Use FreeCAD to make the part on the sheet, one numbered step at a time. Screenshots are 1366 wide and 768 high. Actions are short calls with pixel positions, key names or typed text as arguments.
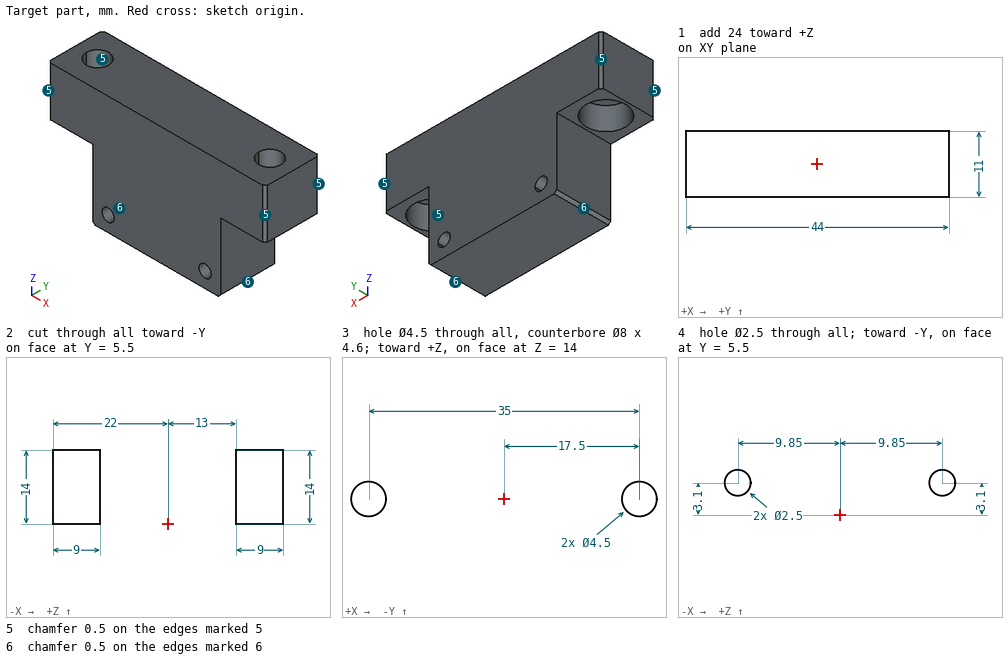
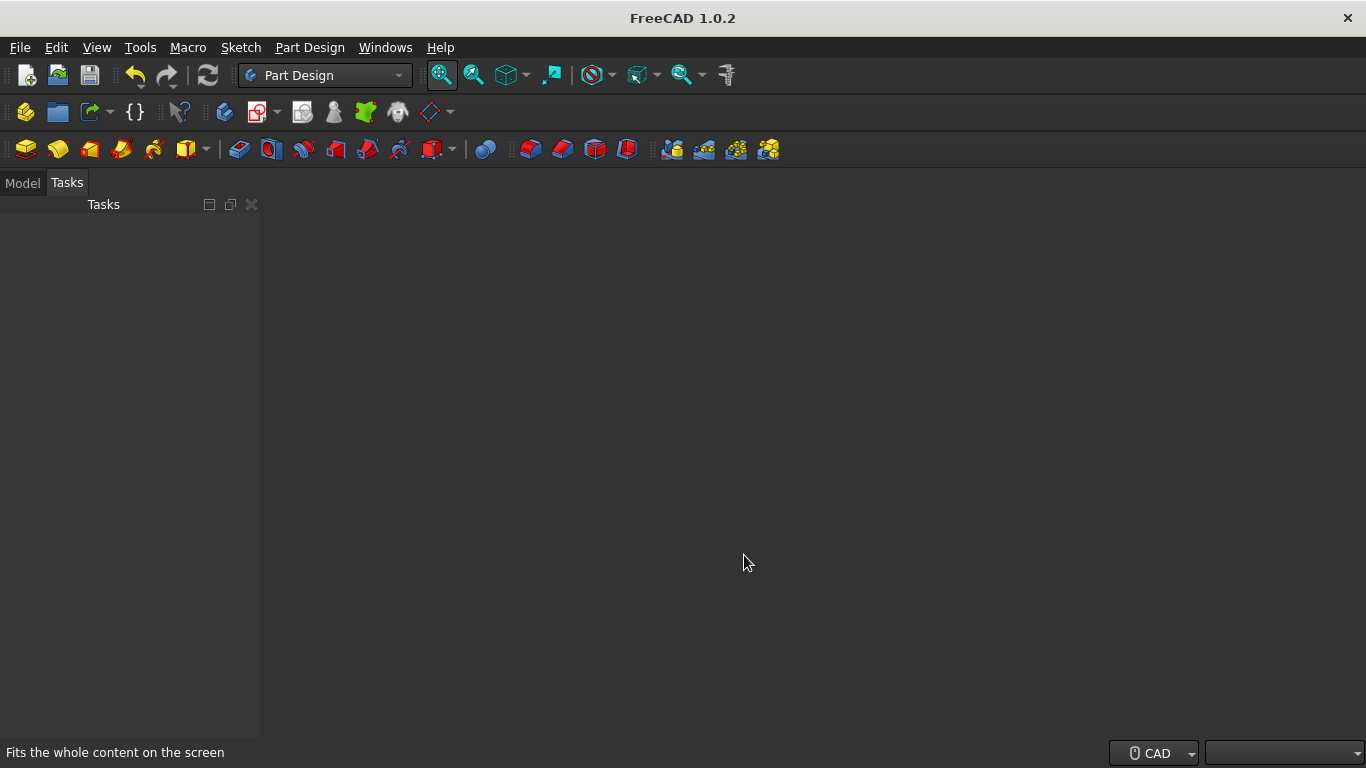
click(26, 76)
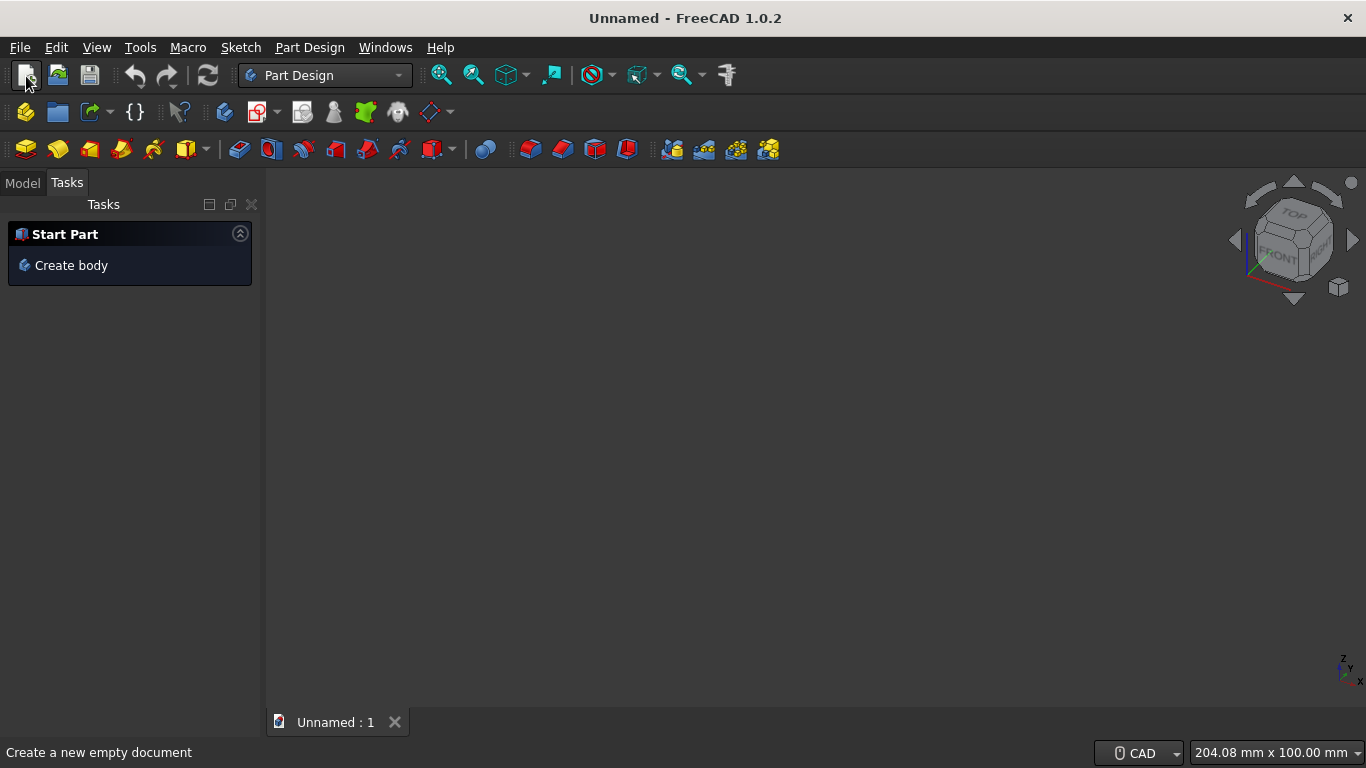
click(258, 112)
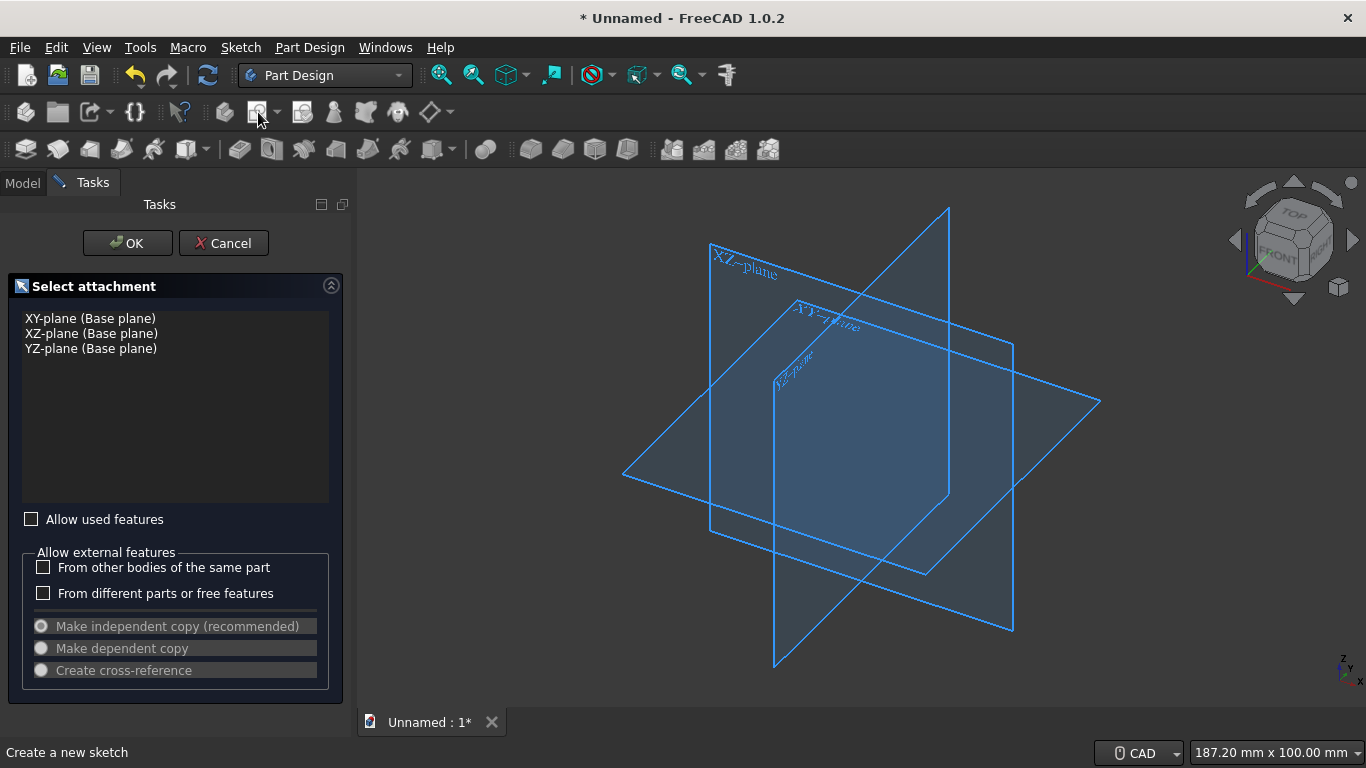
click(82, 318)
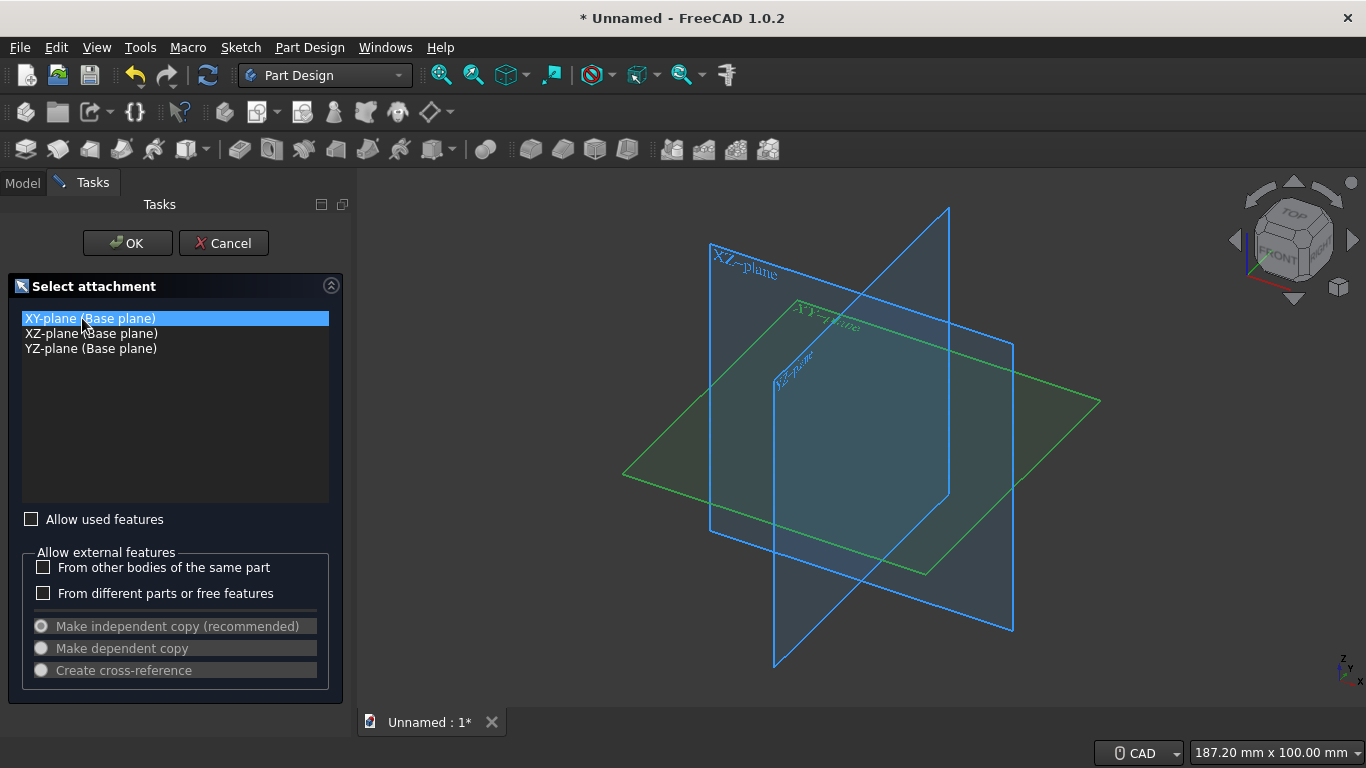
click(128, 243)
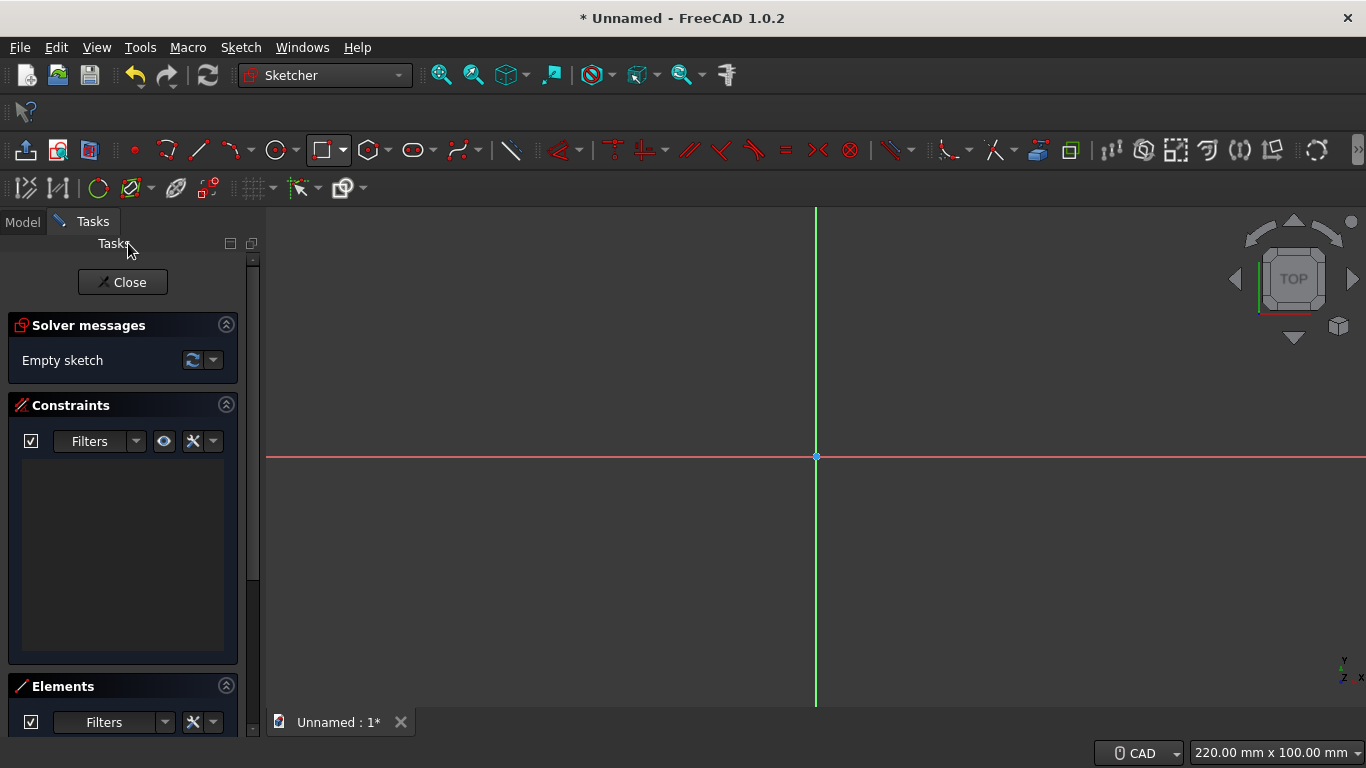
scroll(856, 457, up, 5)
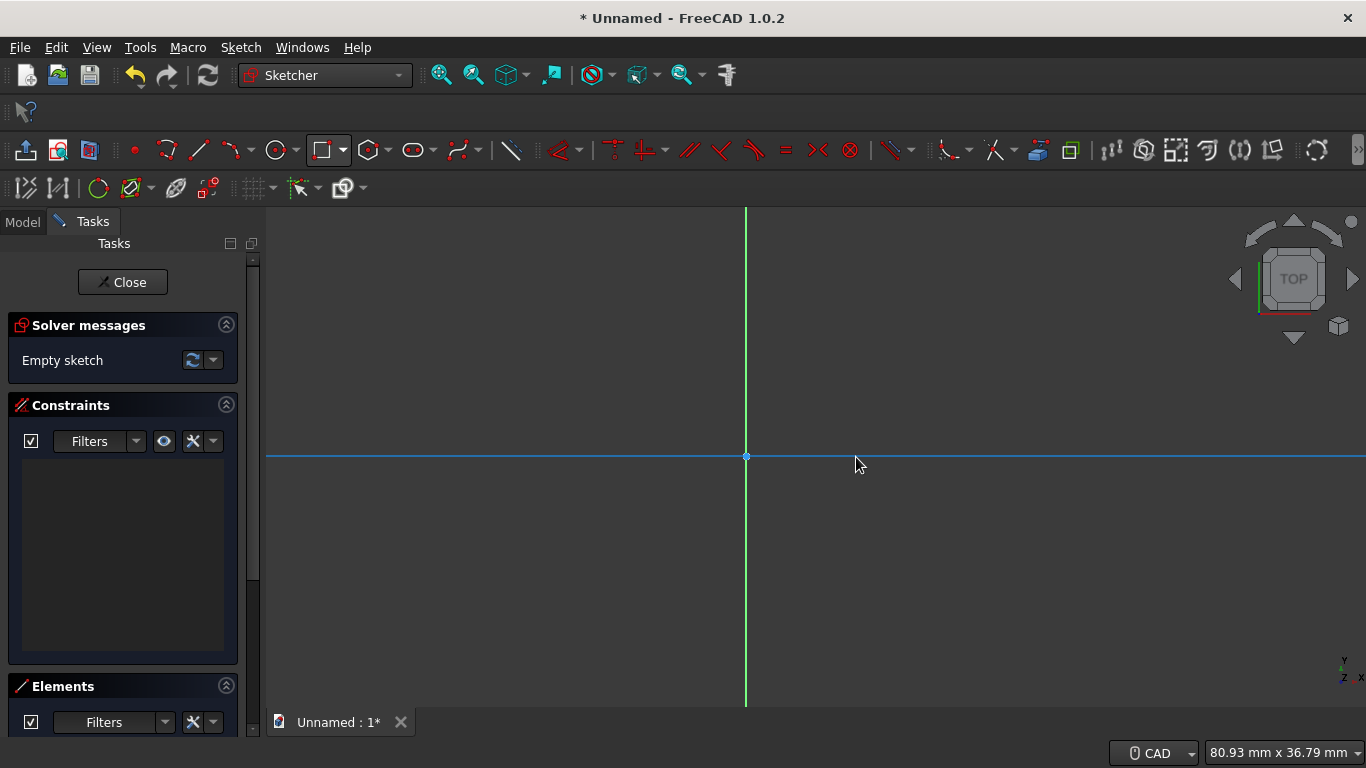
click(346, 150)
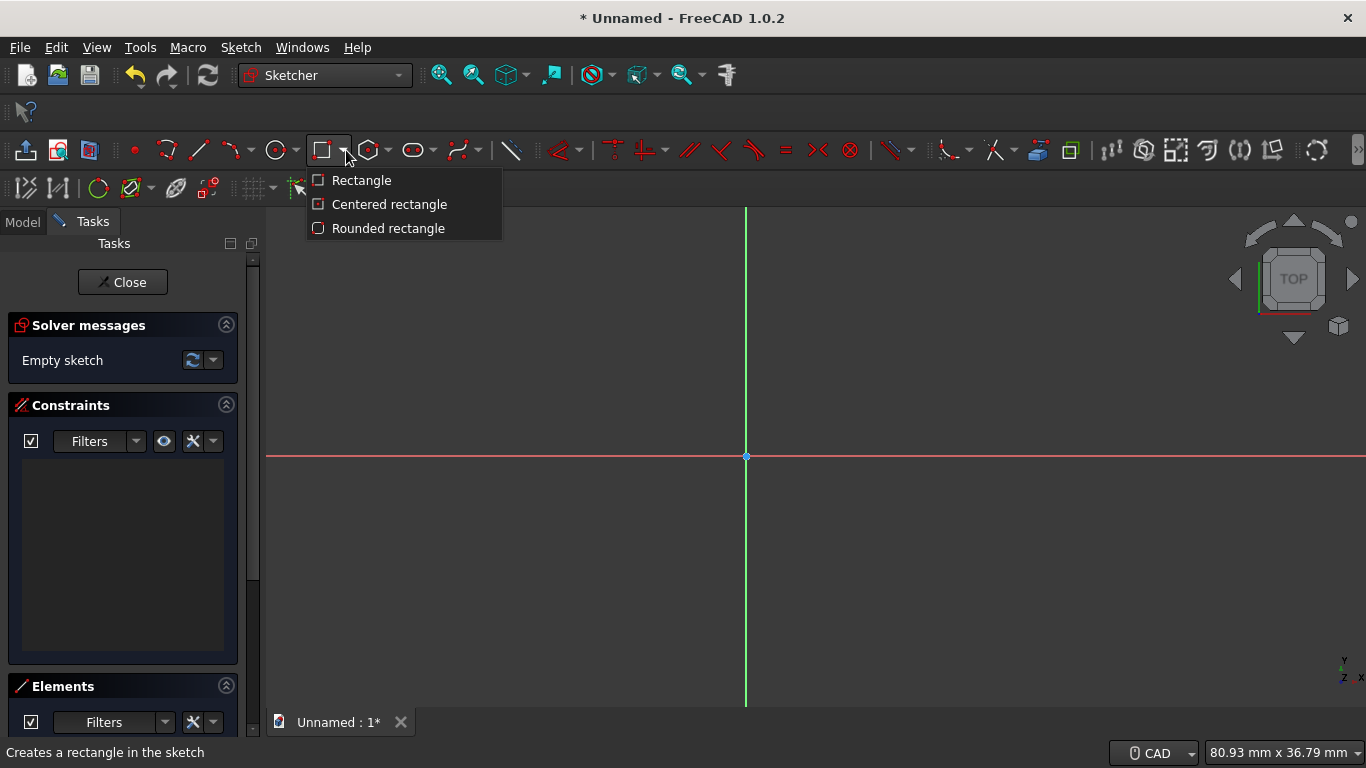
click(404, 204)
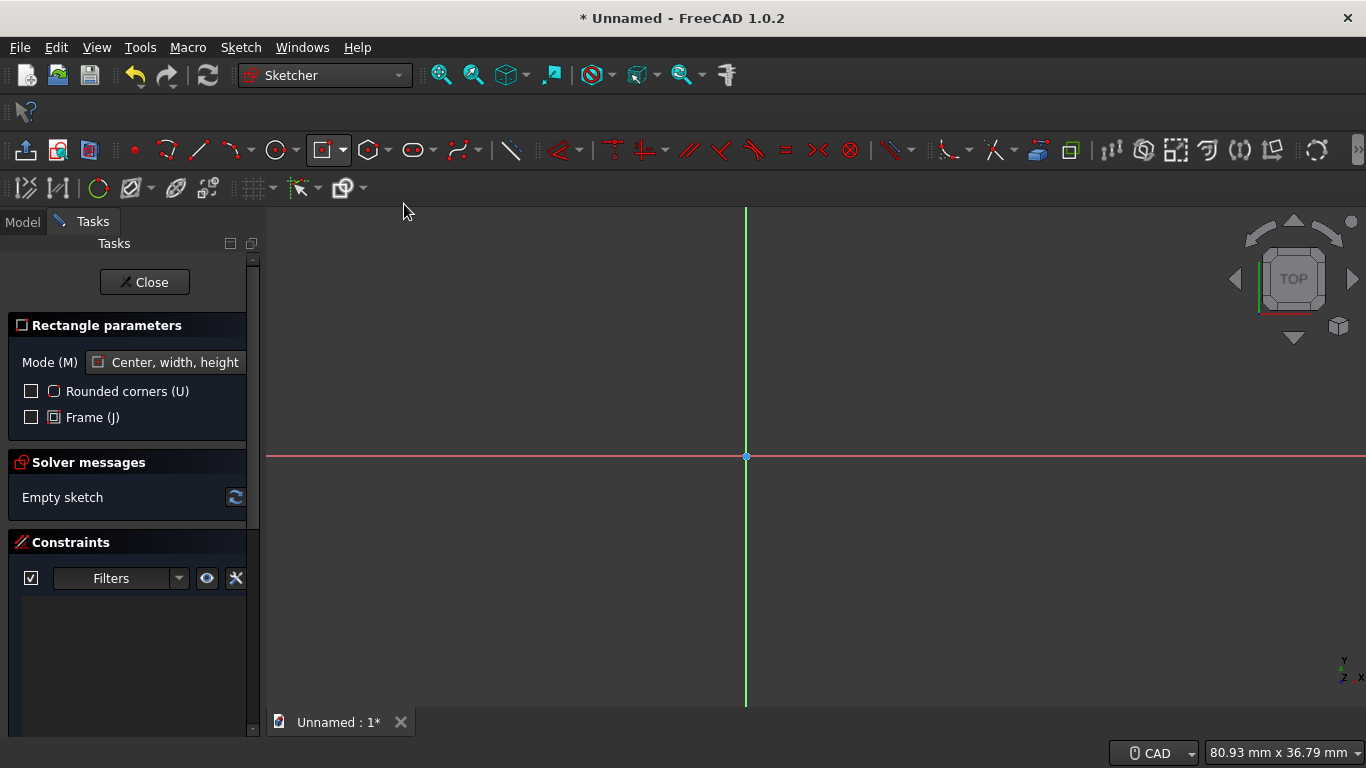
click(746, 456)
move(1045, 381)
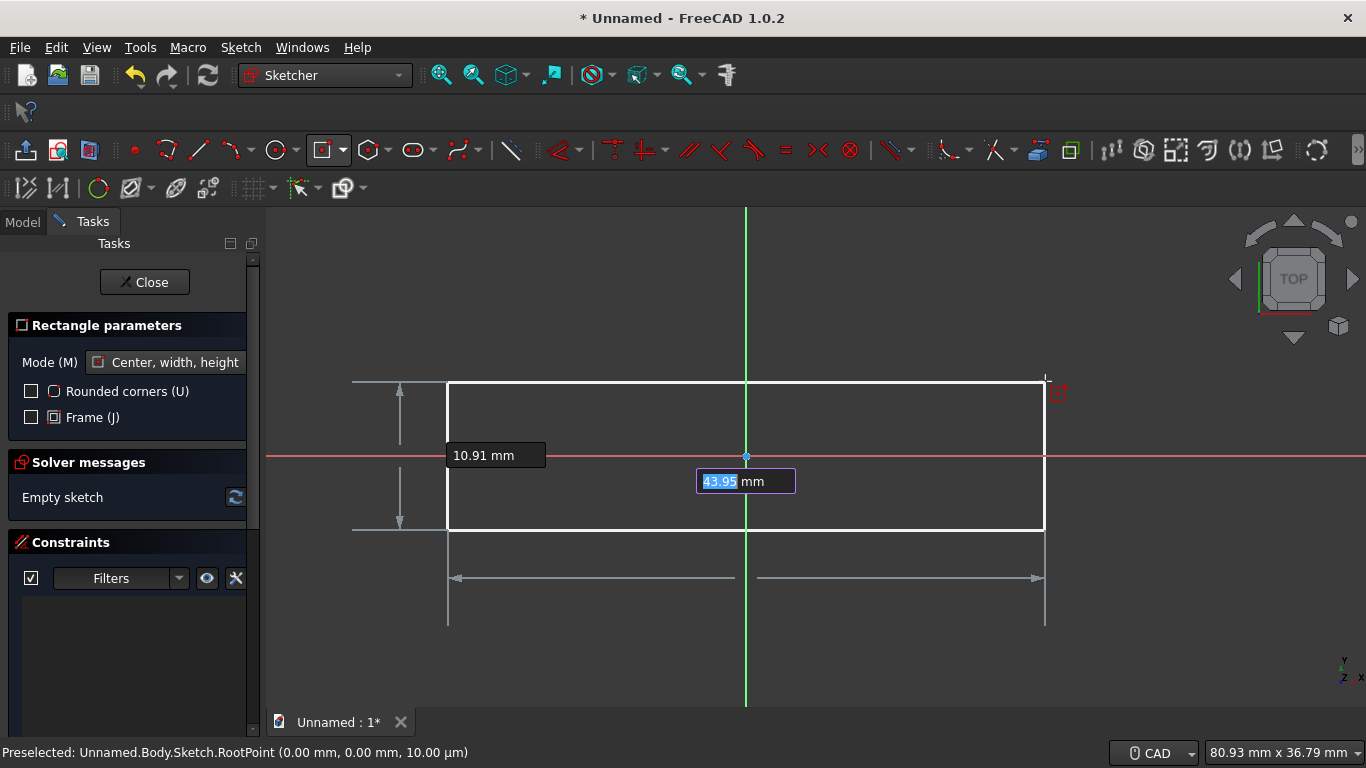
text(44)
key(Tab)
text(11)
key(Return)
key(Escape)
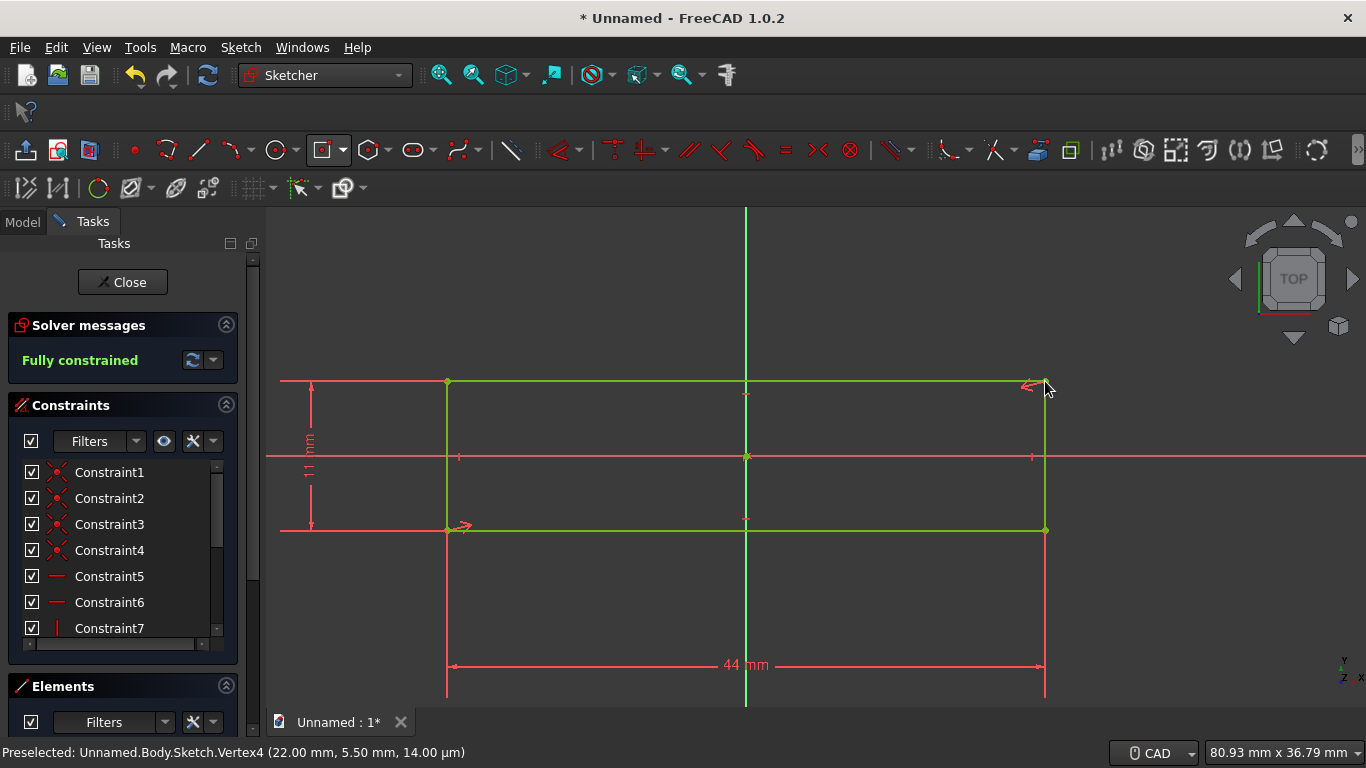
click(123, 282)